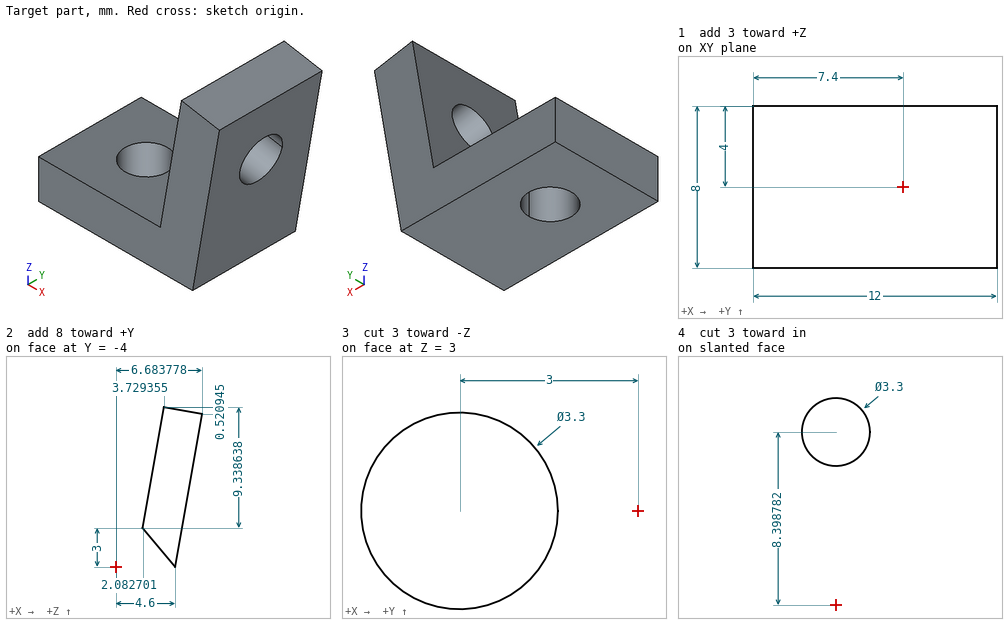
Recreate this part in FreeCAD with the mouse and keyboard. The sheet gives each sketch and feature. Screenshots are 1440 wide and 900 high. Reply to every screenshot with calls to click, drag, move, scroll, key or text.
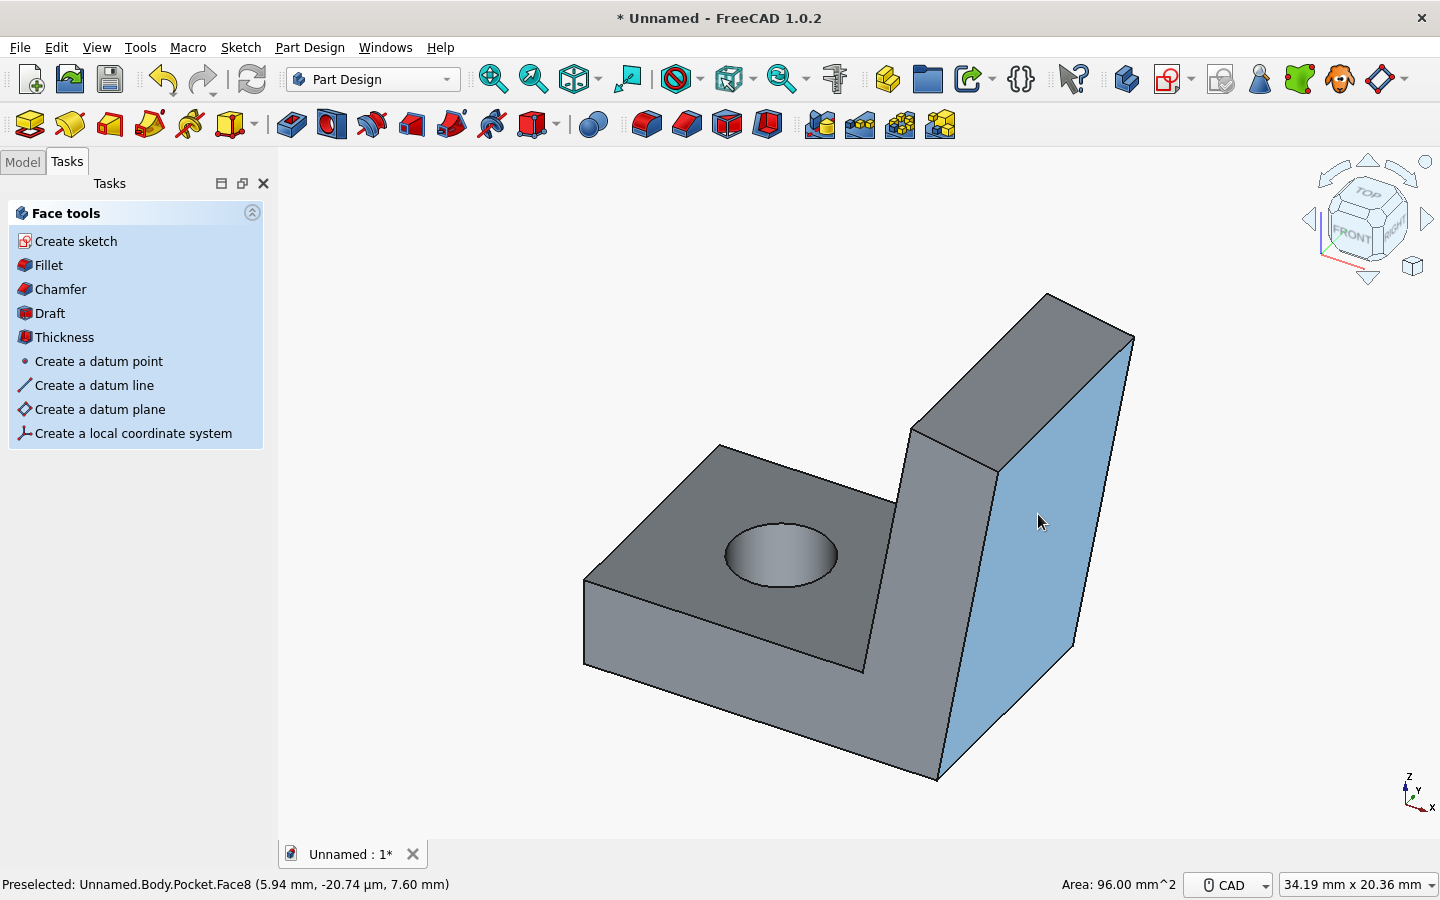
click(1168, 80)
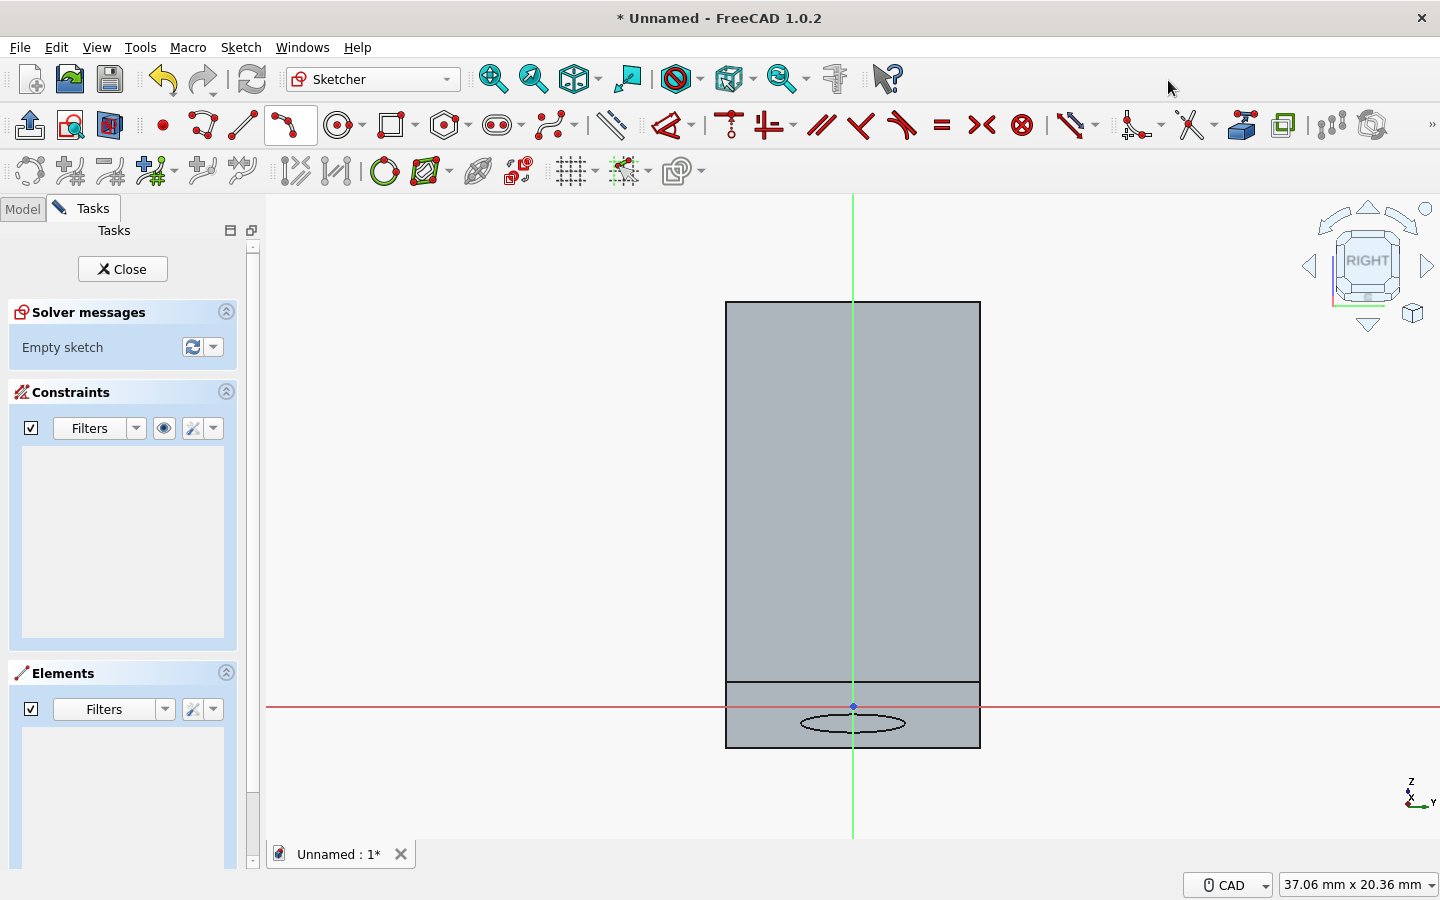
scroll(875, 416, up, 7)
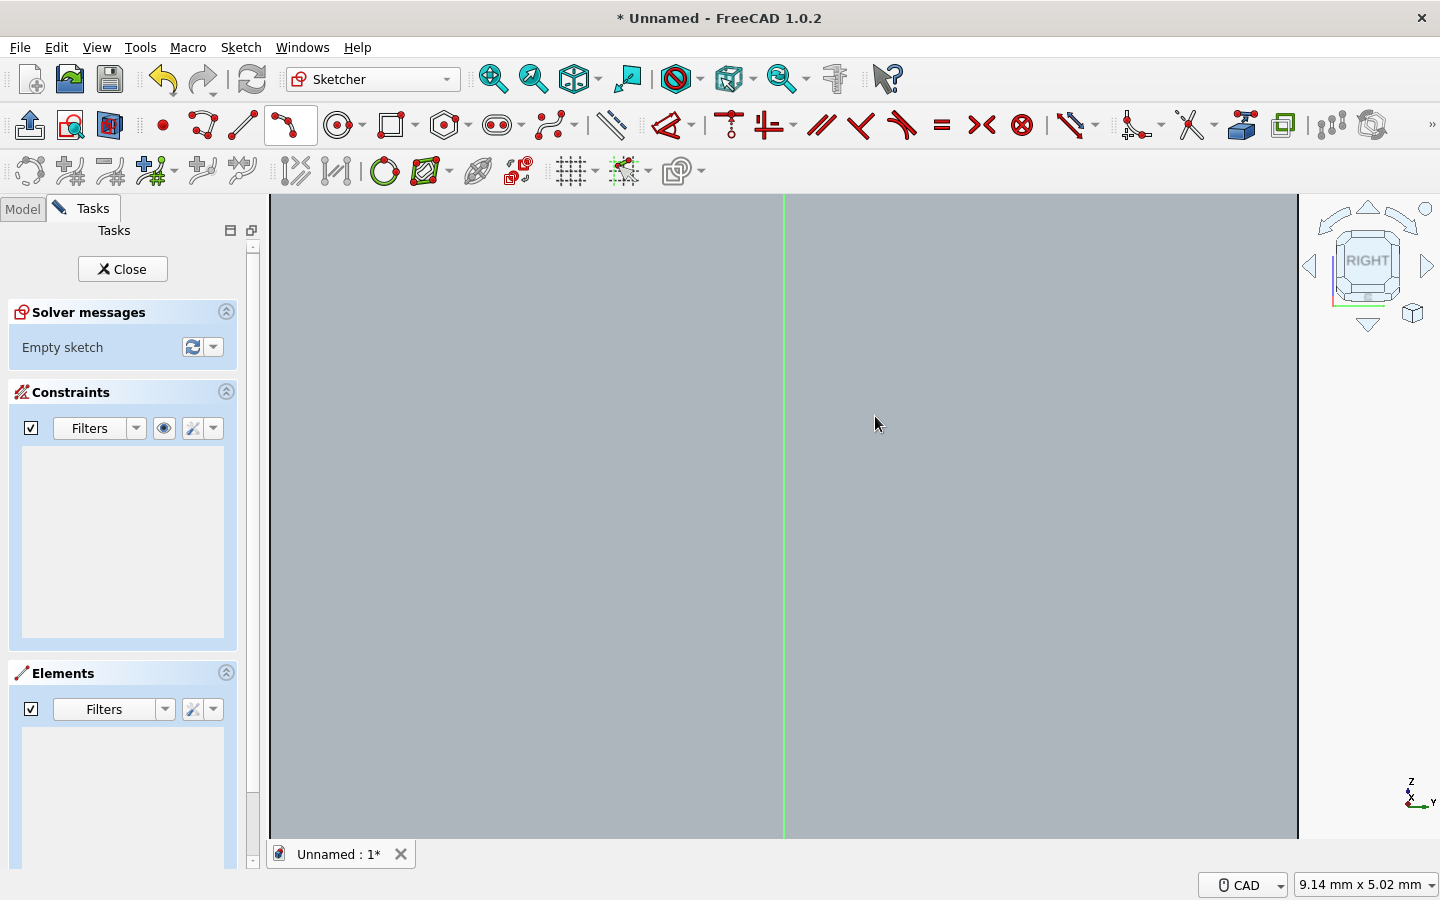
click(338, 126)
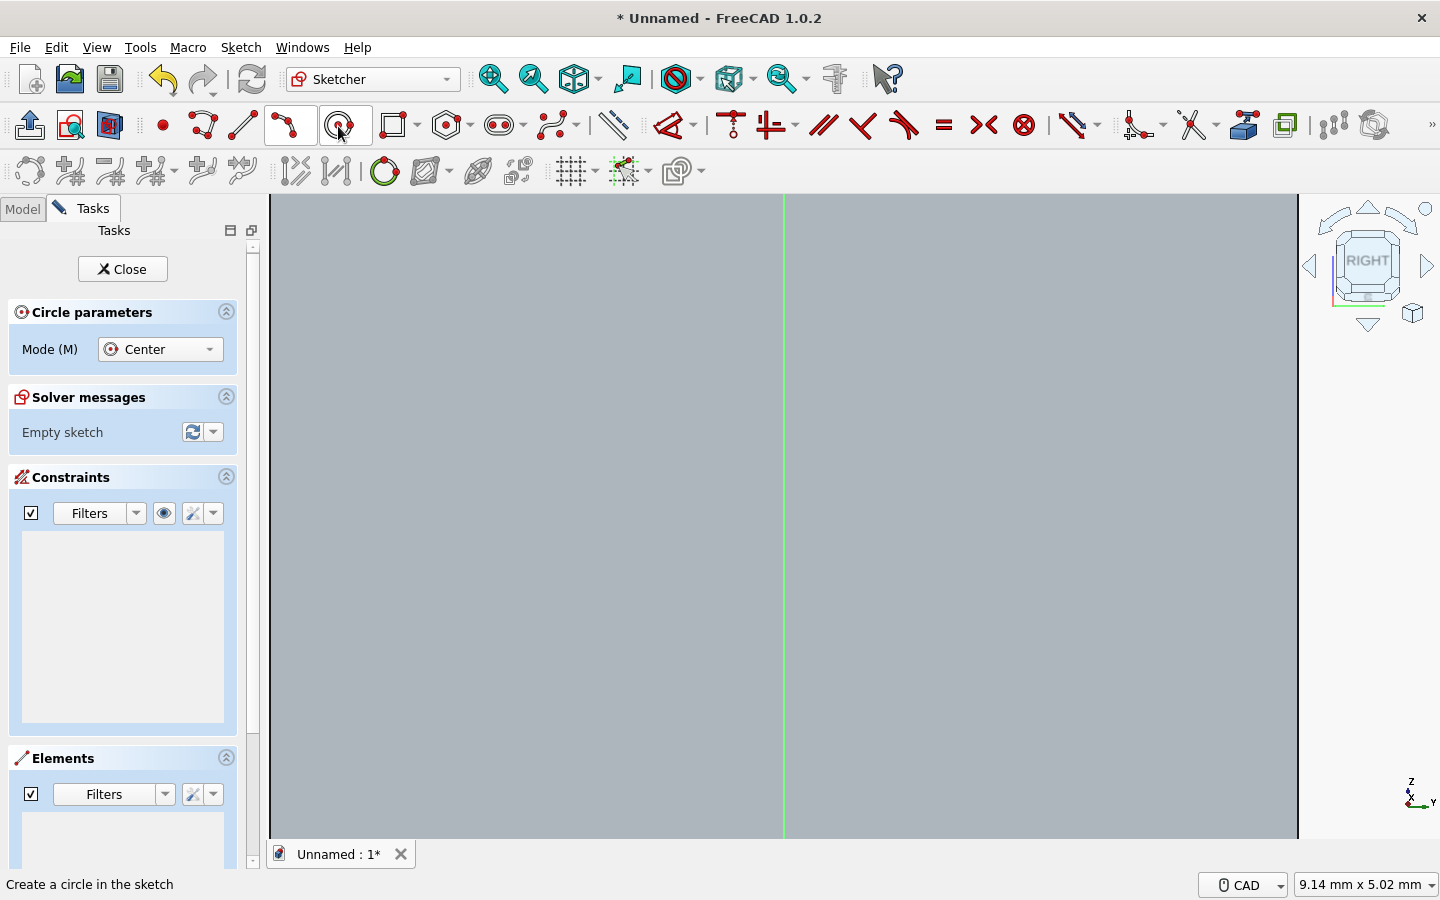
click(784, 516)
click(934, 366)
key(Escape)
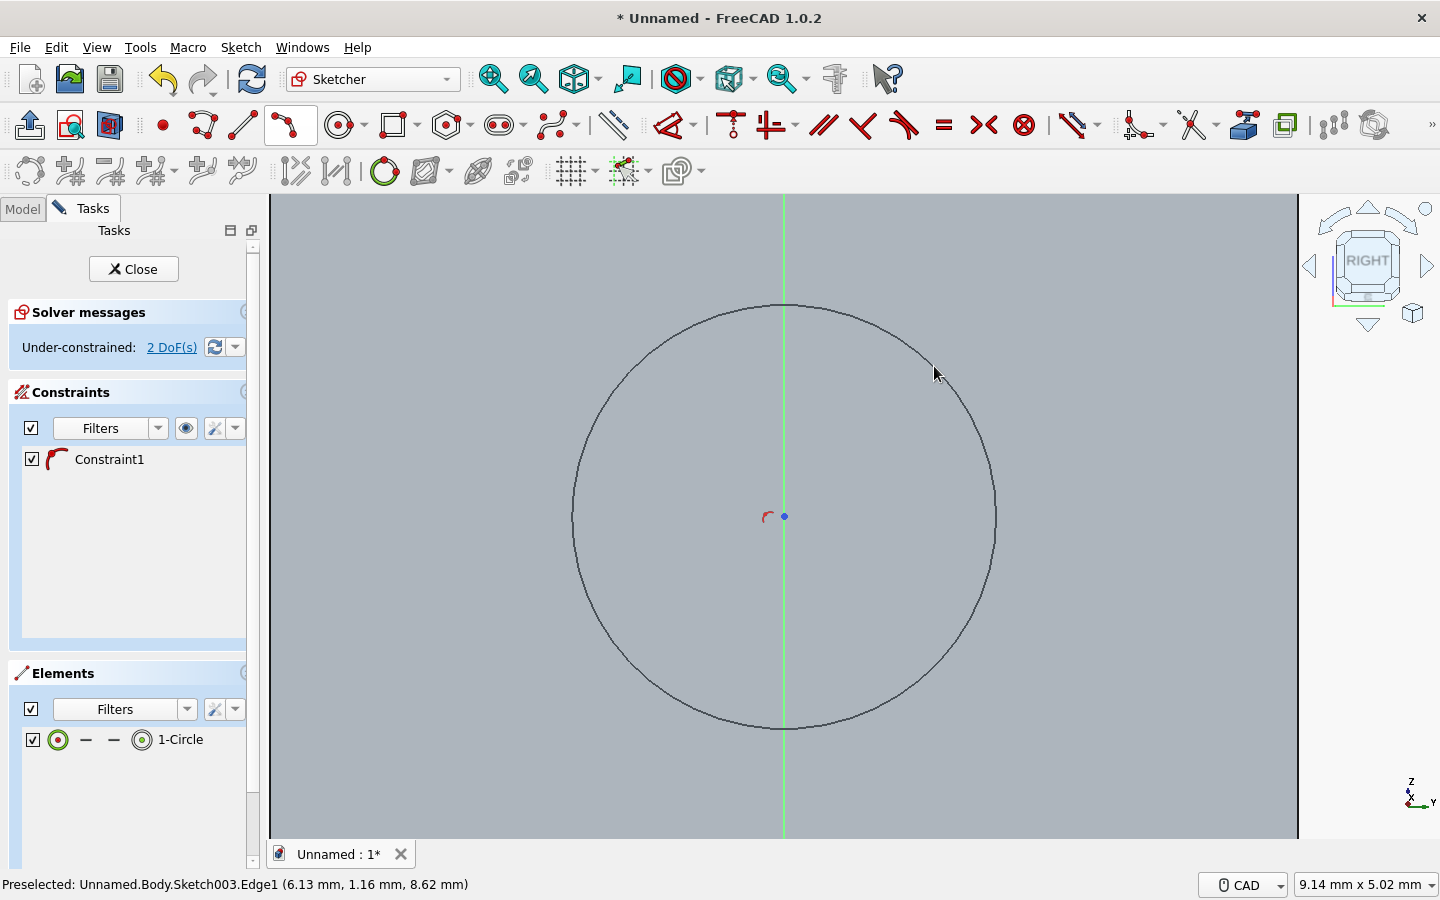
click(668, 126)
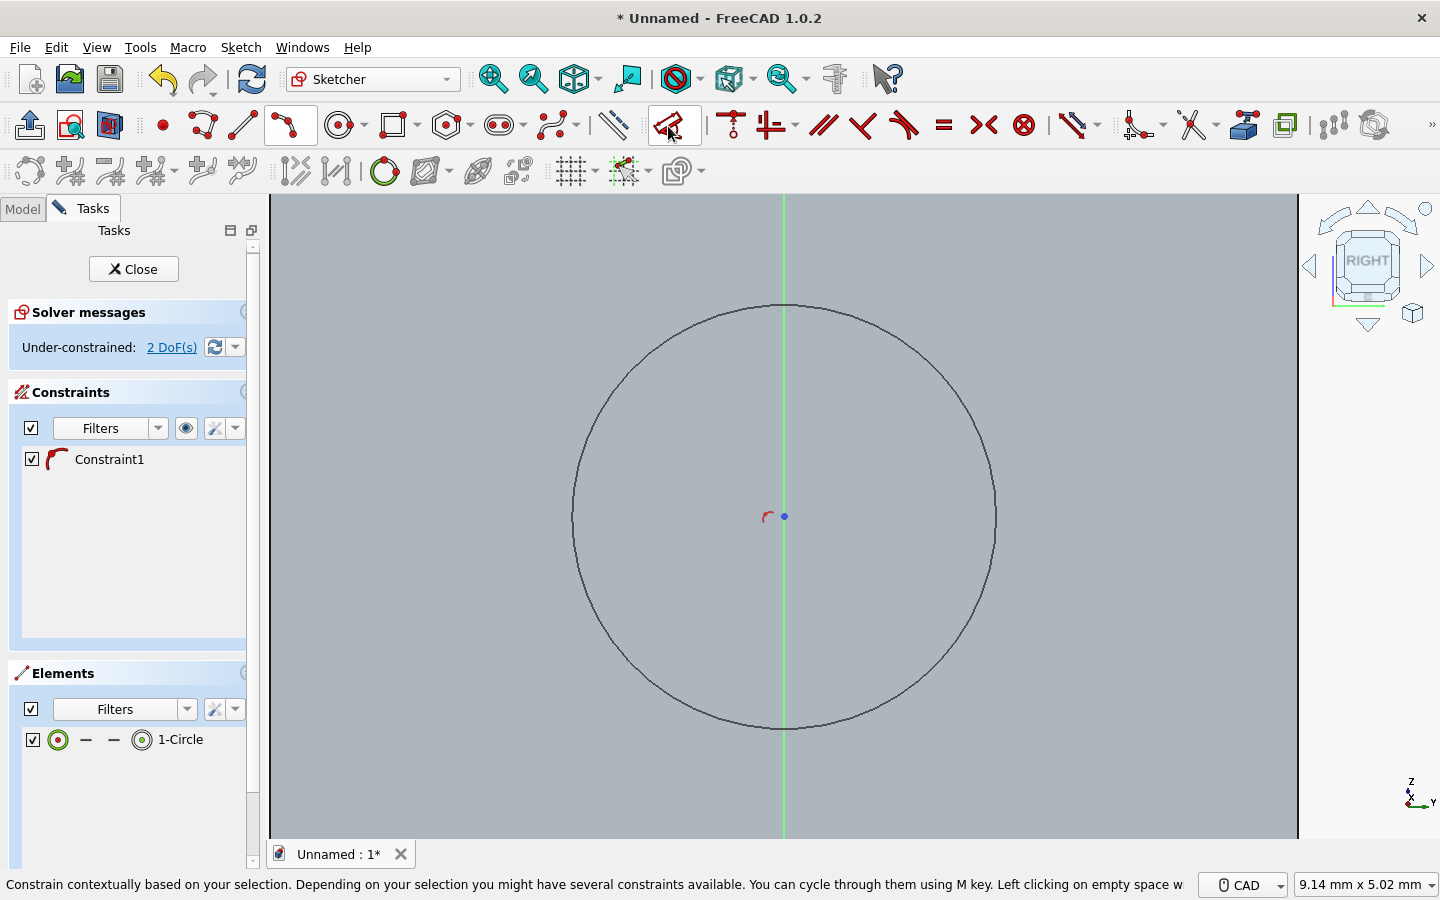
click(934, 367)
click(957, 344)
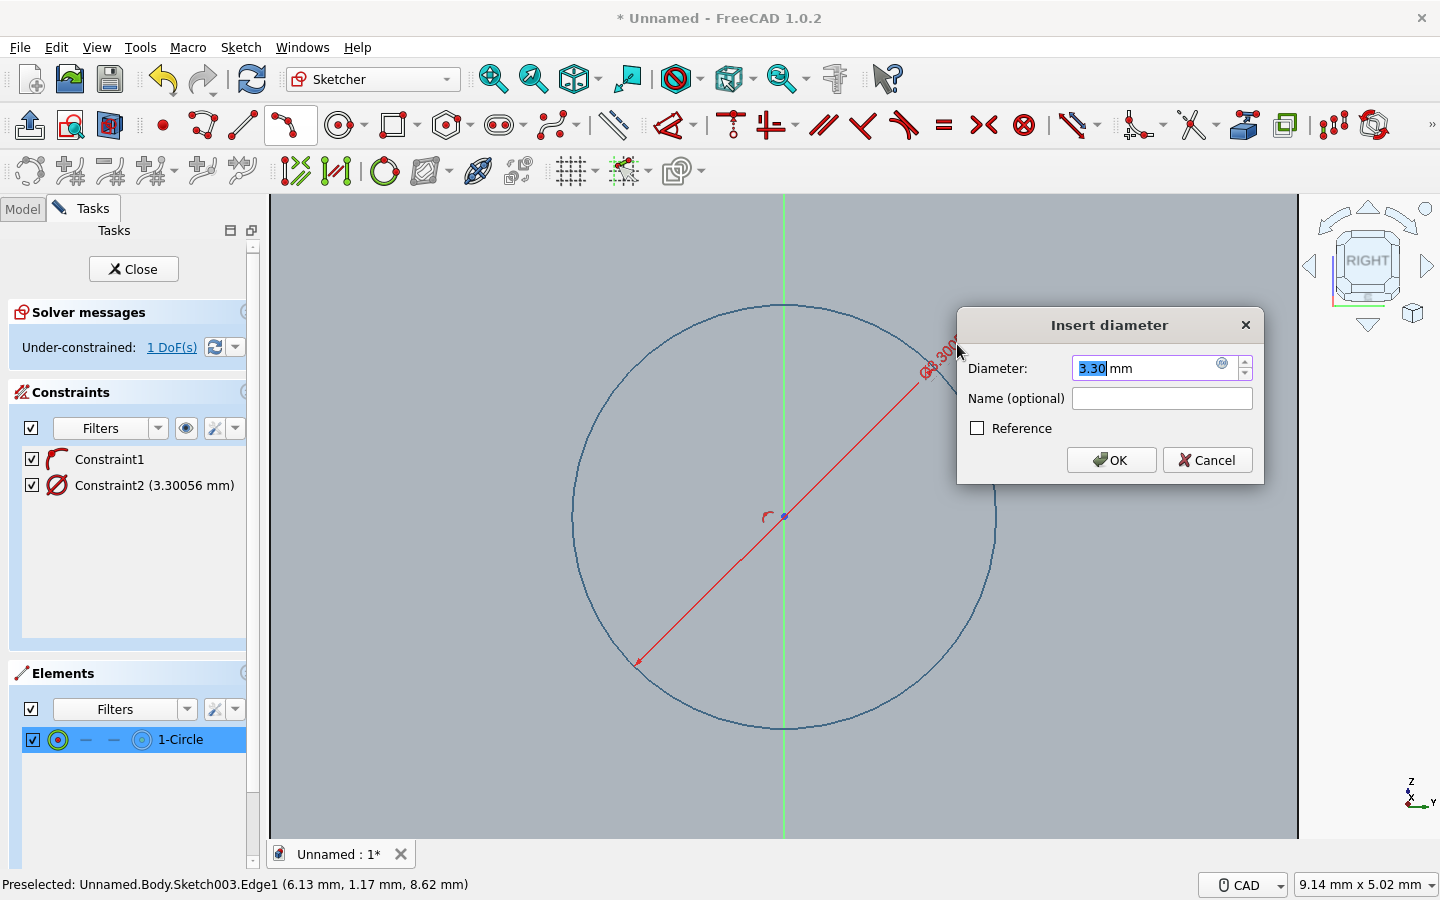
text(3.3)
key(Return)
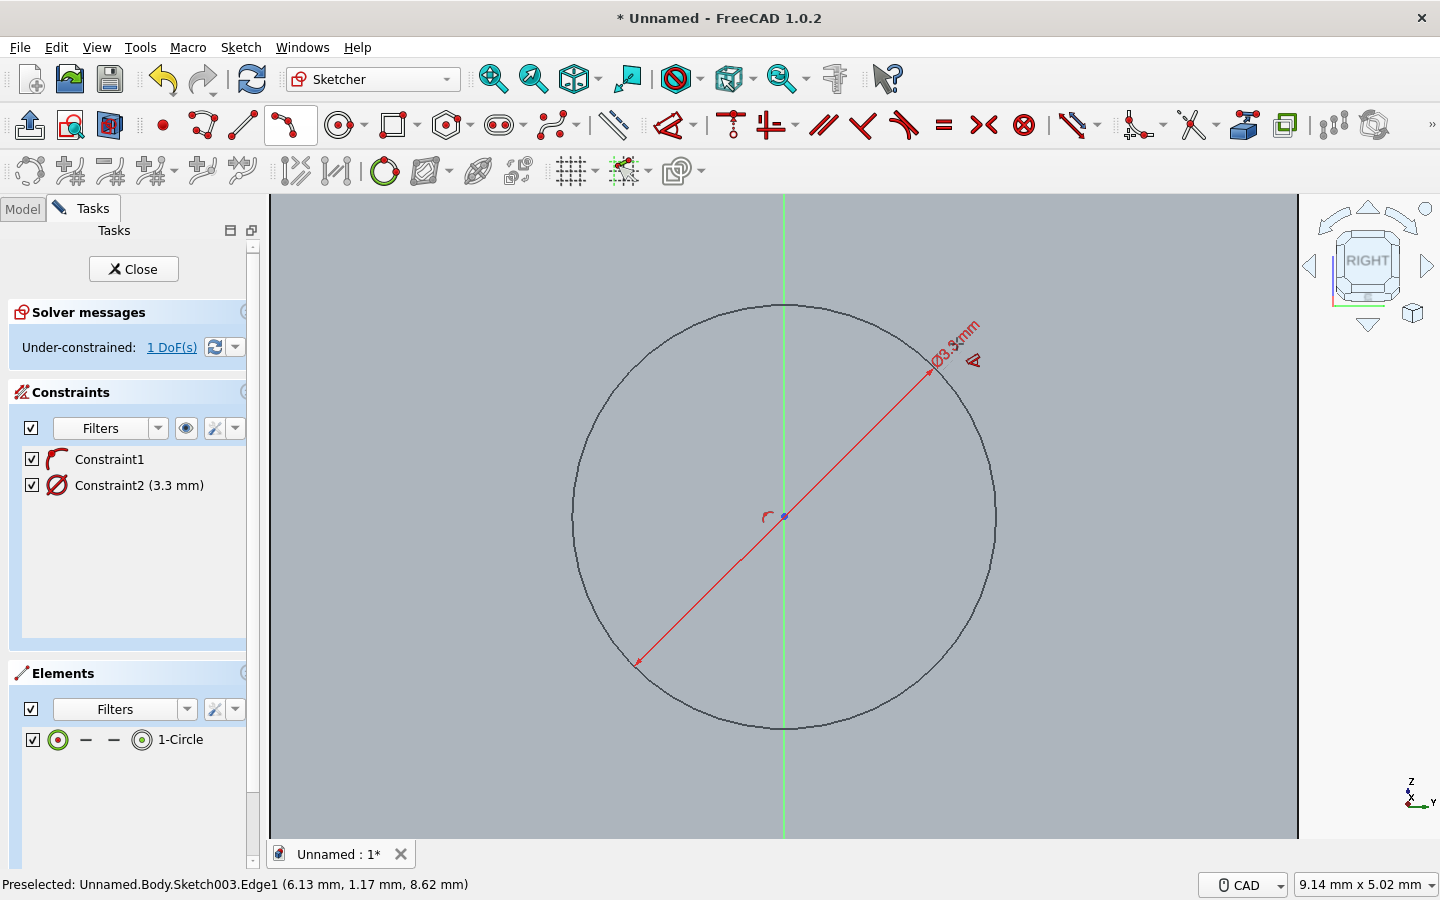
click(784, 517)
click(818, 664)